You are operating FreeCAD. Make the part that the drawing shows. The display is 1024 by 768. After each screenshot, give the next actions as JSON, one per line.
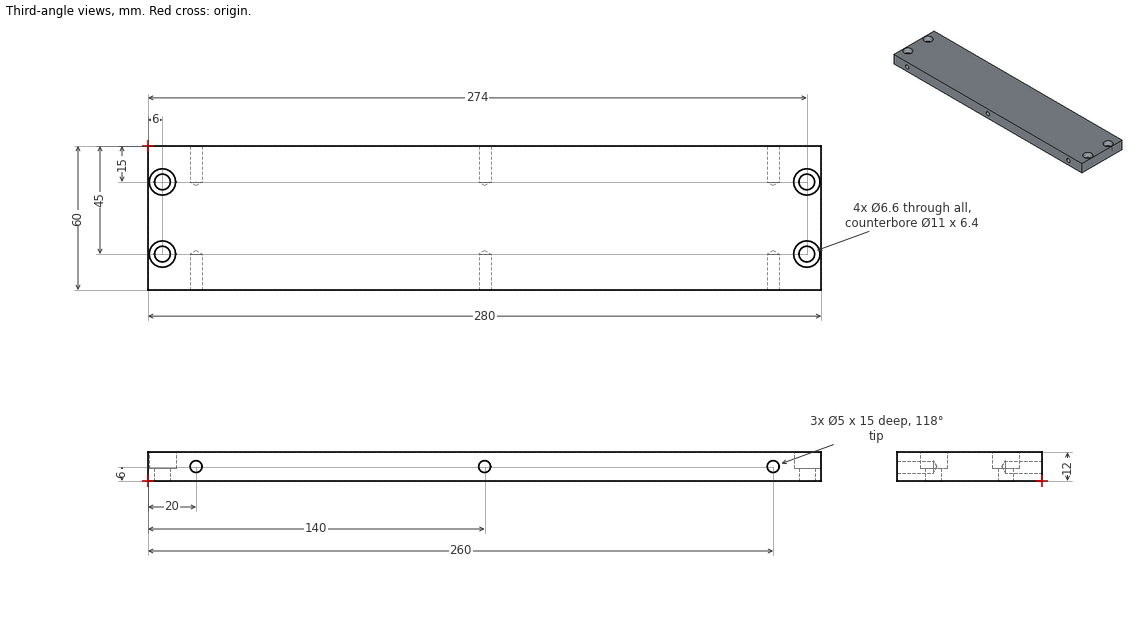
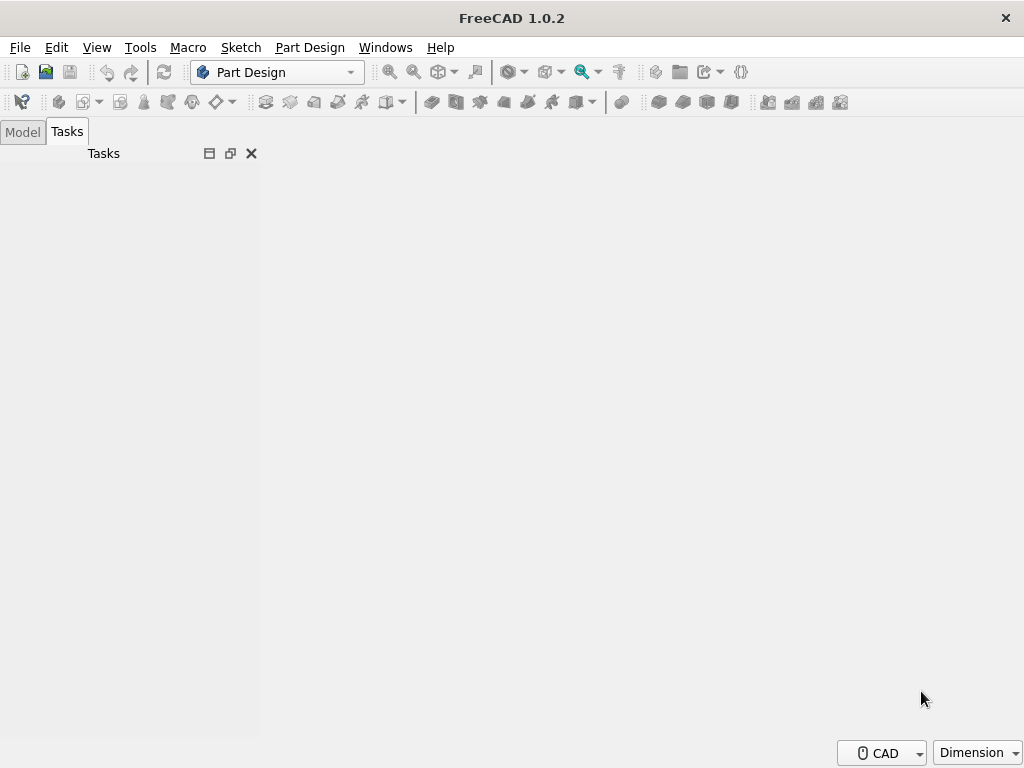
{"action": "left_click", "coordinate": [22, 72]}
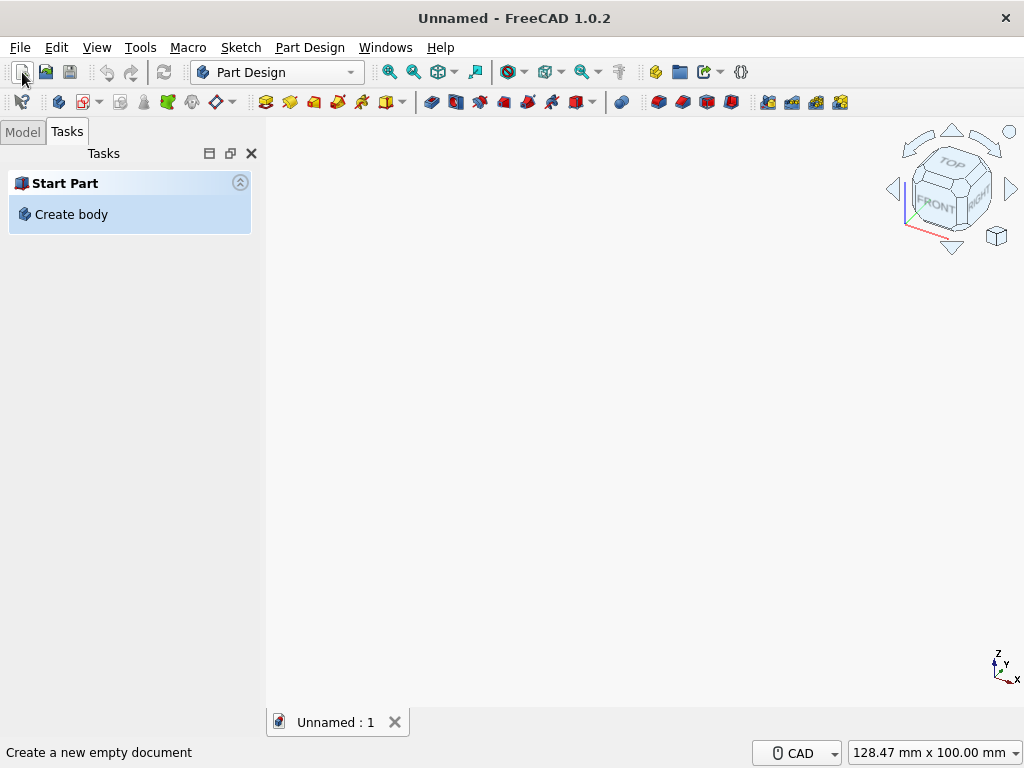
{"action": "left_click", "coordinate": [84, 102]}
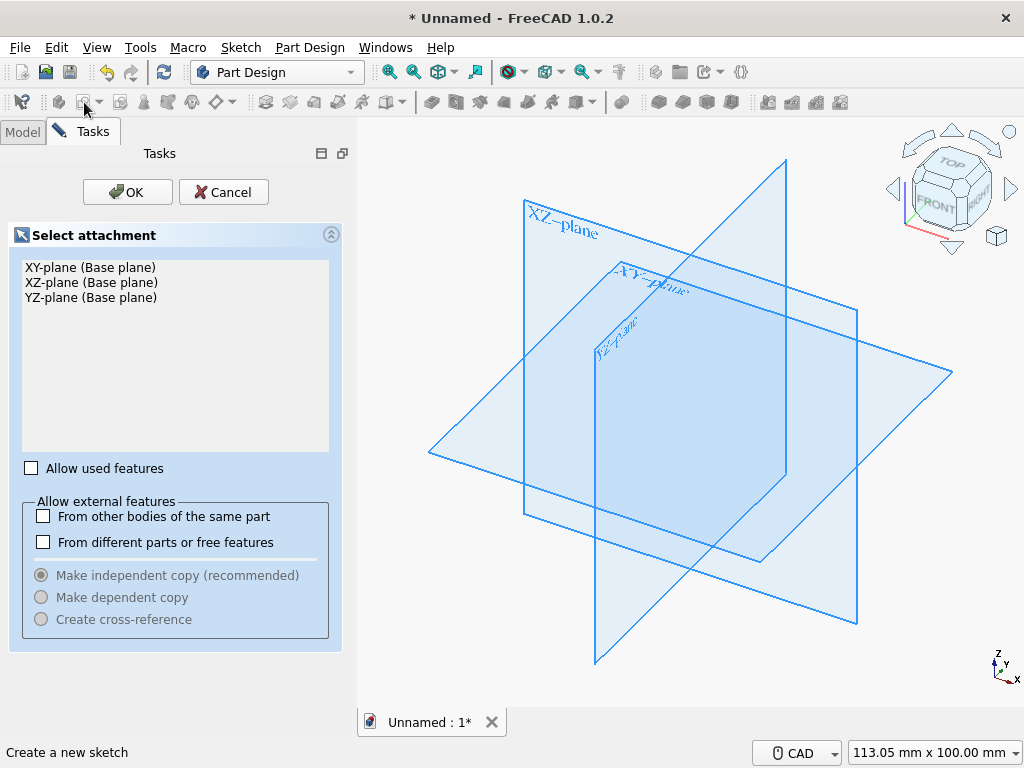
{"action": "left_click", "coordinate": [82, 268]}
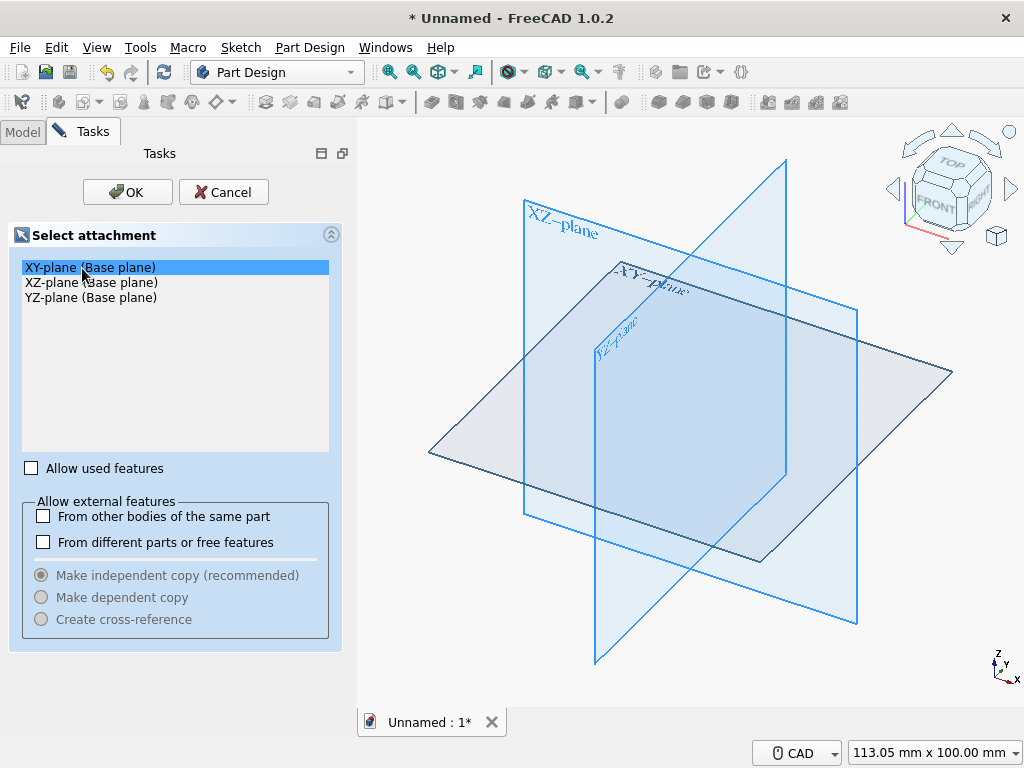
{"action": "left_click", "coordinate": [128, 192]}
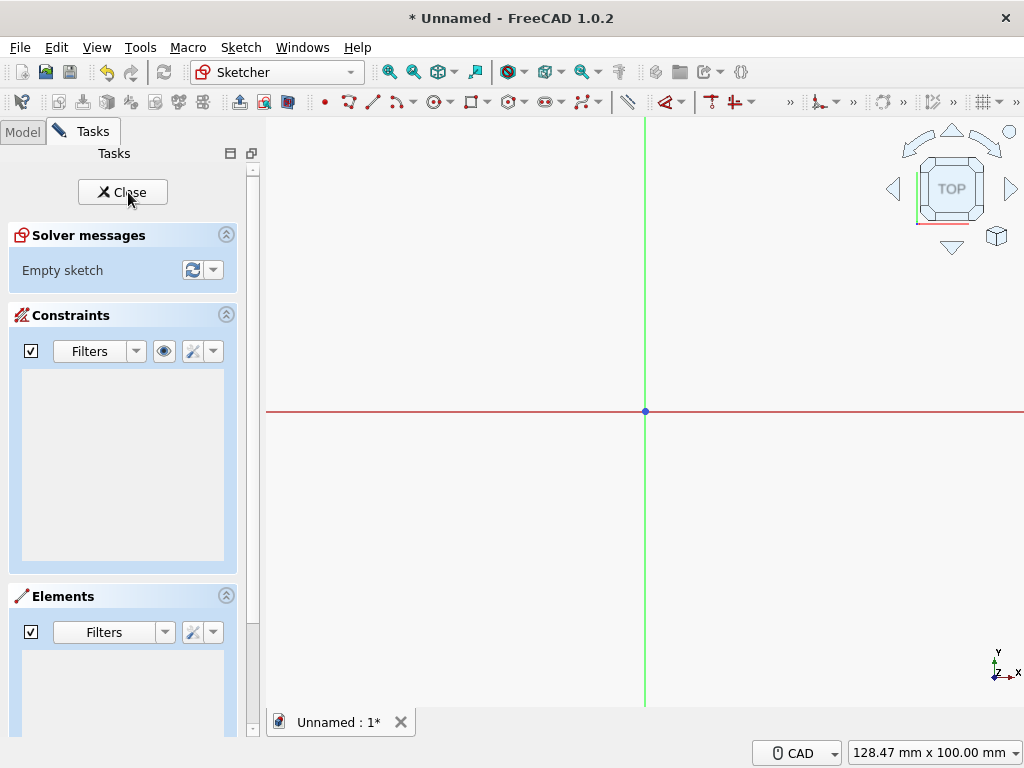
{"action": "scroll", "coordinate": [294, 354], "scroll_direction": "down", "scroll_amount": 7}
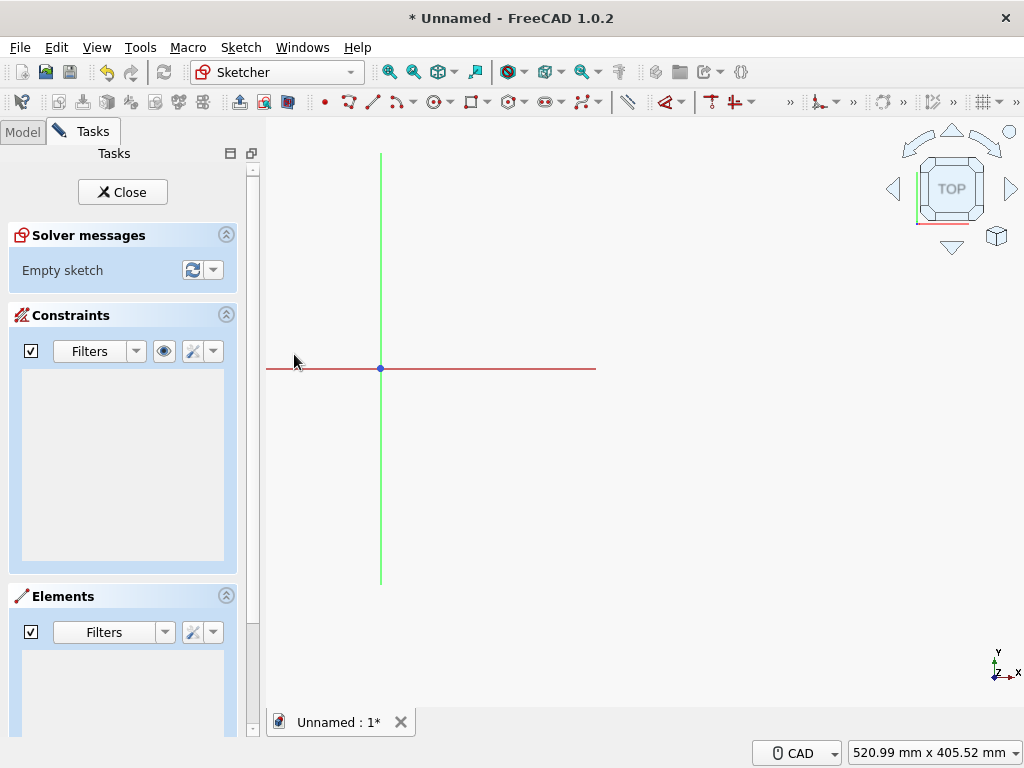
{"action": "left_click", "coordinate": [472, 102]}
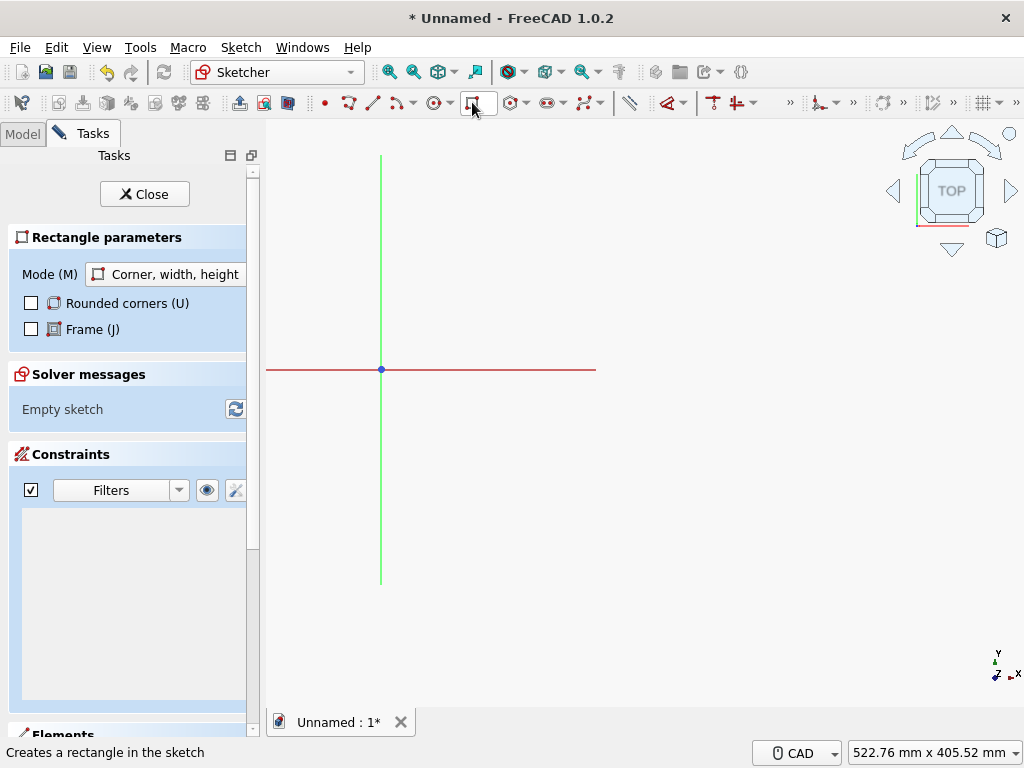
{"action": "left_click", "coordinate": [381, 370]}
{"action": "left_click", "coordinate": [787, 457]}
{"action": "key", "text": "Escape"}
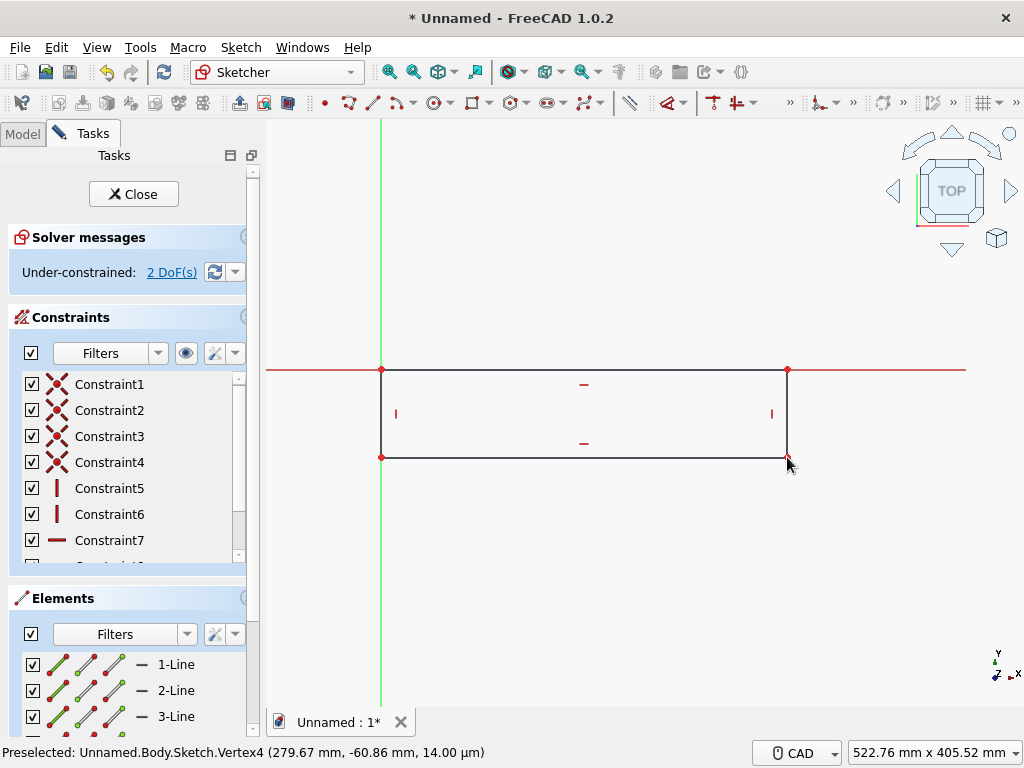
{"action": "left_click", "coordinate": [668, 104]}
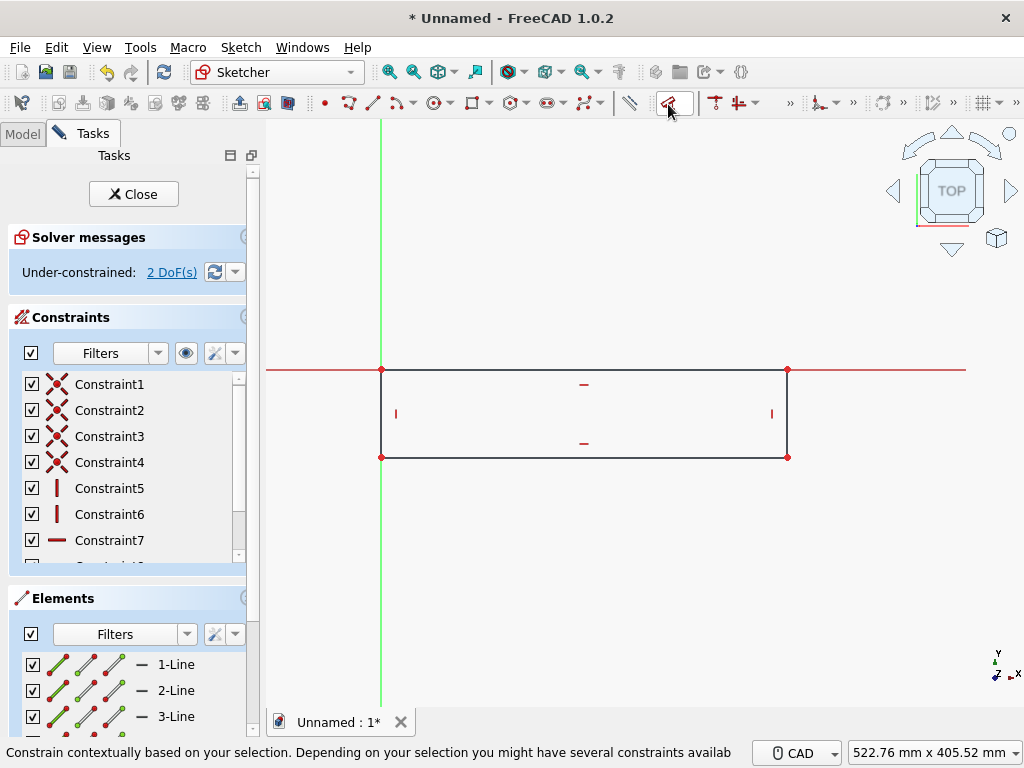
{"action": "left_click", "coordinate": [381, 396]}
{"action": "left_click", "coordinate": [347, 414]}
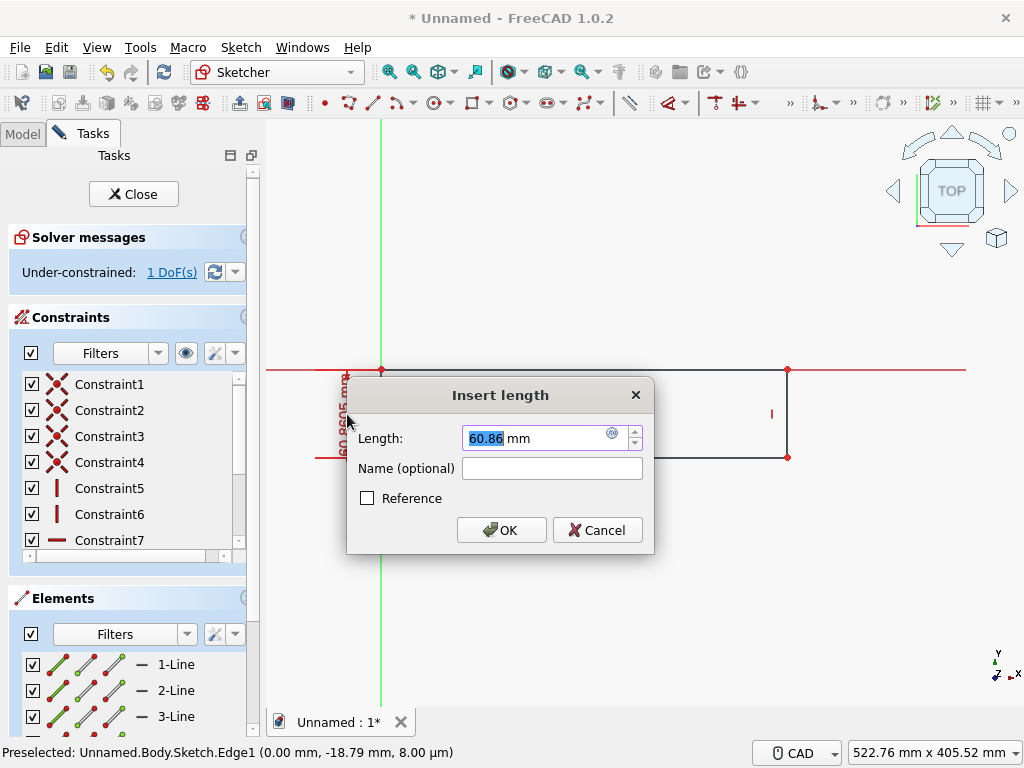
{"action": "type", "text": "60"}
{"action": "key", "text": "Return"}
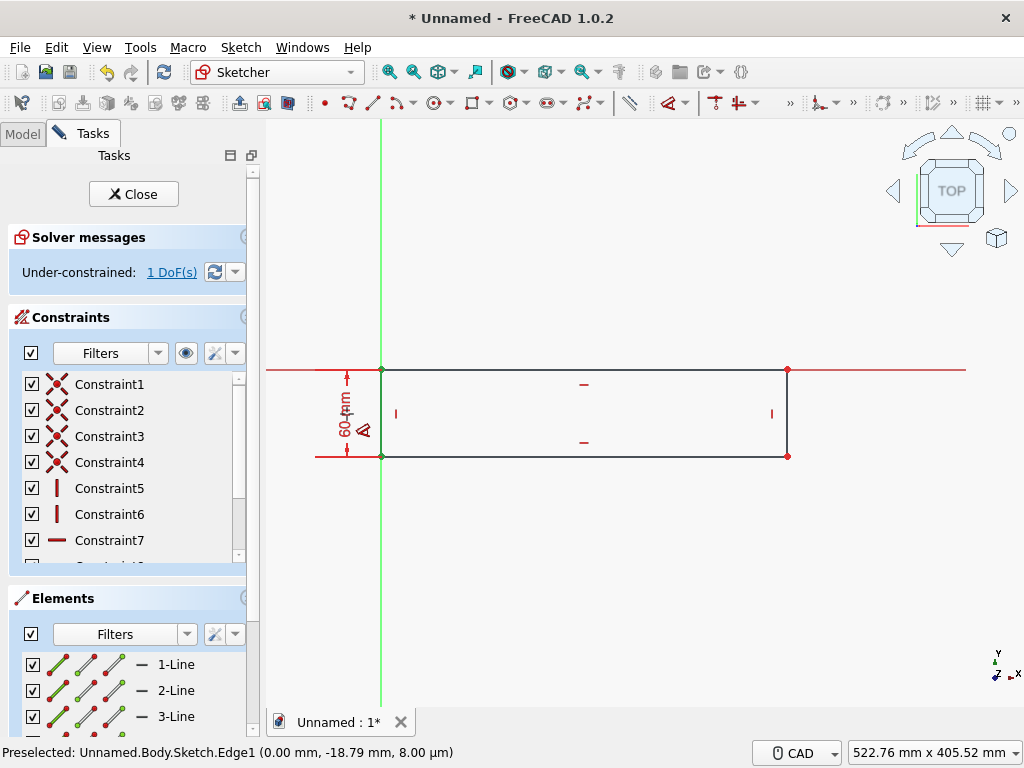
{"action": "left_click", "coordinate": [503, 457]}
{"action": "left_click", "coordinate": [584, 491]}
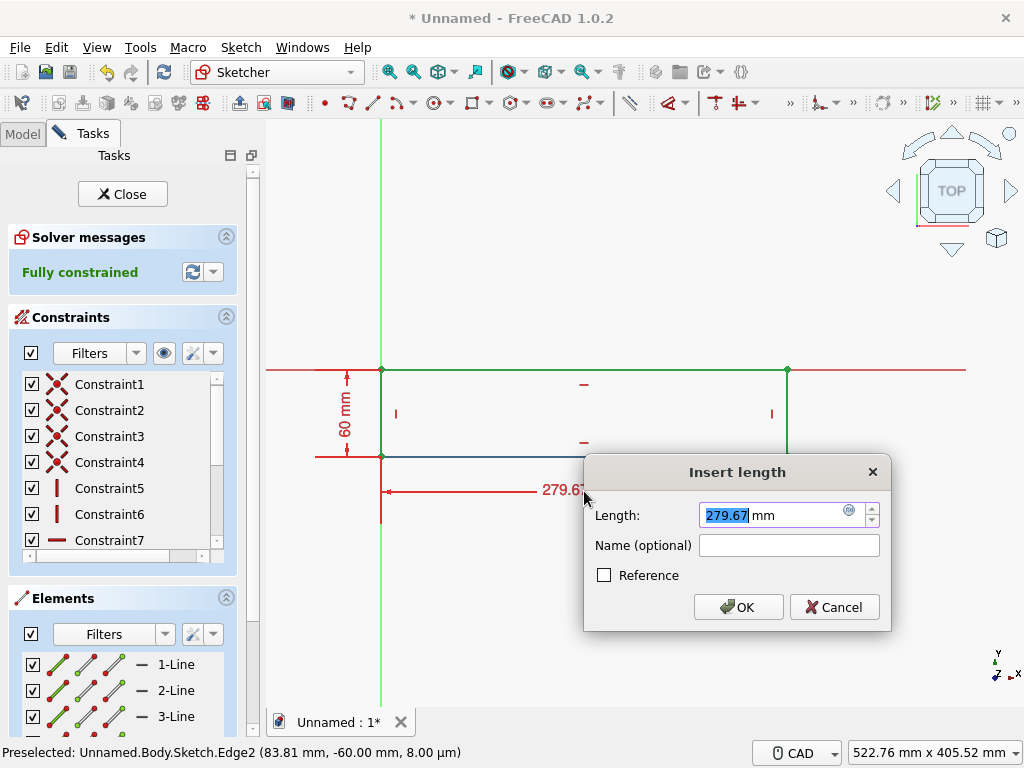
{"action": "type", "text": "280"}
{"action": "key", "text": "Return"}
{"action": "key", "text": "Escape"}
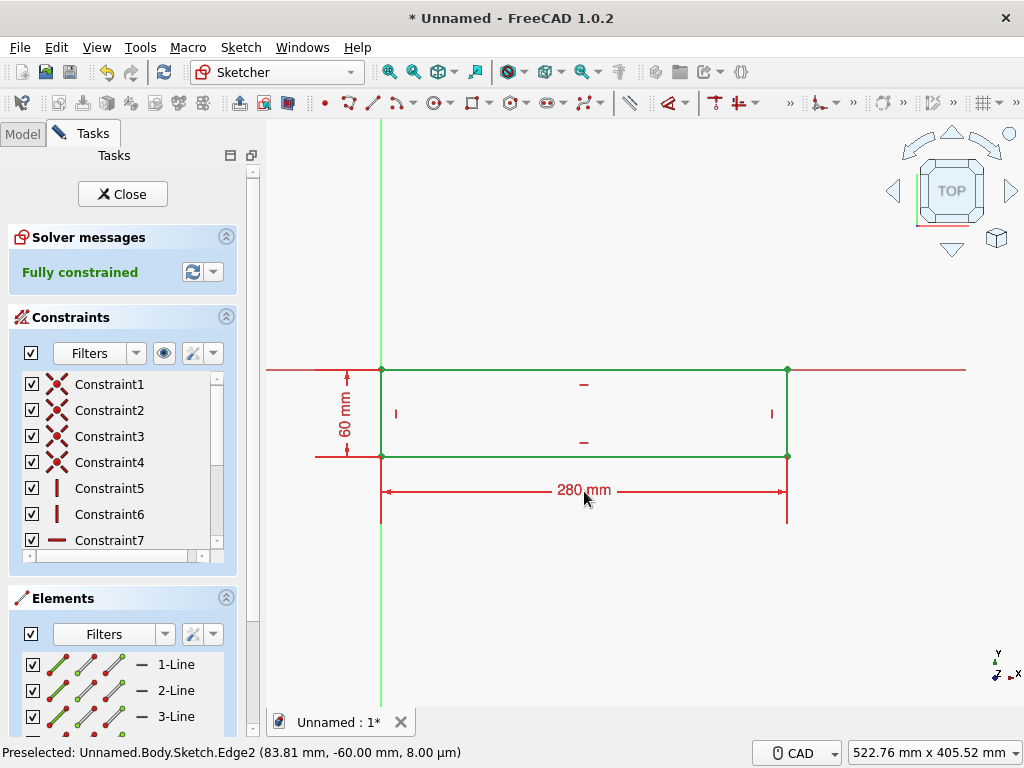
{"action": "left_click", "coordinate": [123, 194]}